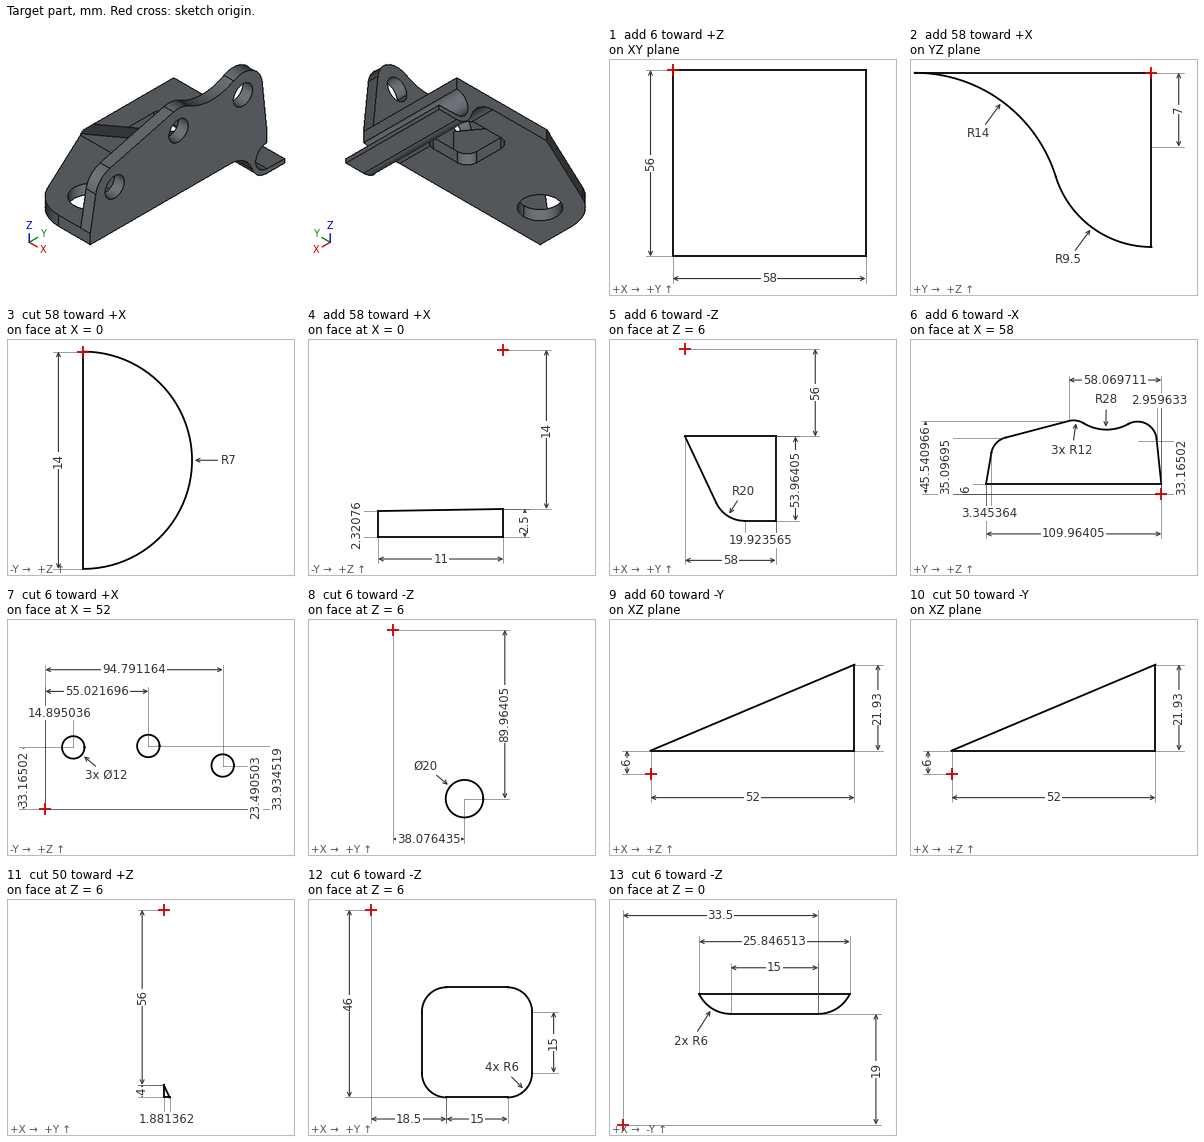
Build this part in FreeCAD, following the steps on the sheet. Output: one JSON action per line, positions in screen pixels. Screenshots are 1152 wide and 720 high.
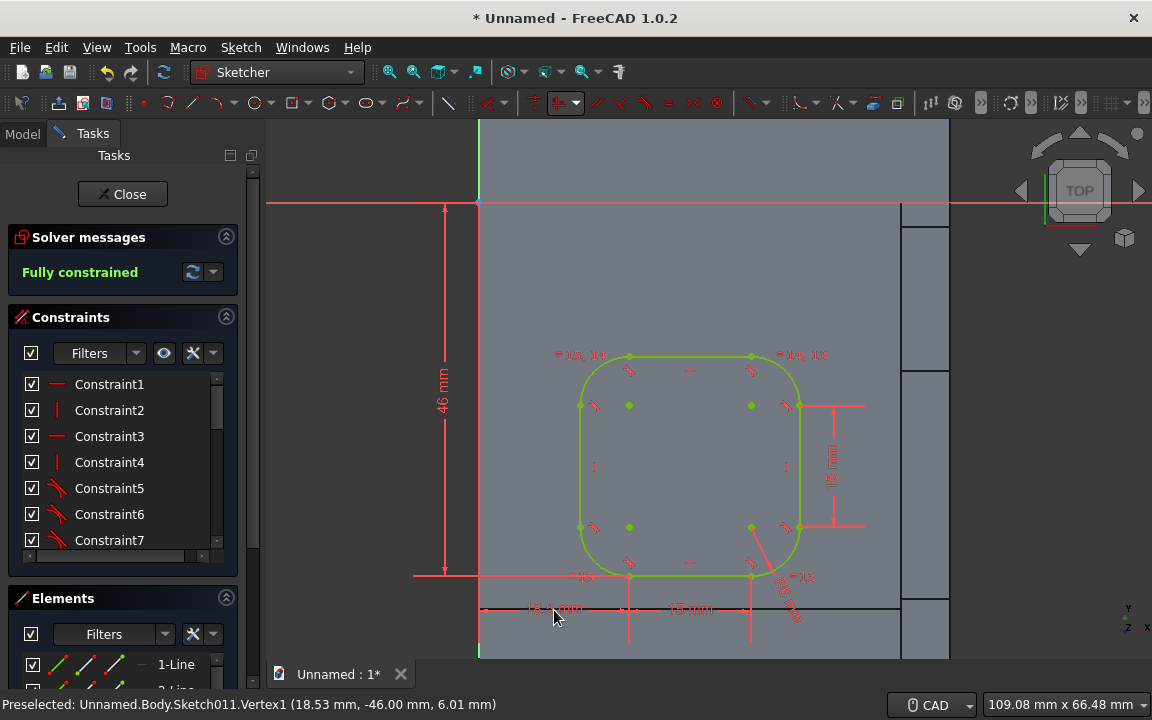
{"action": "left_click", "coordinate": [123, 194]}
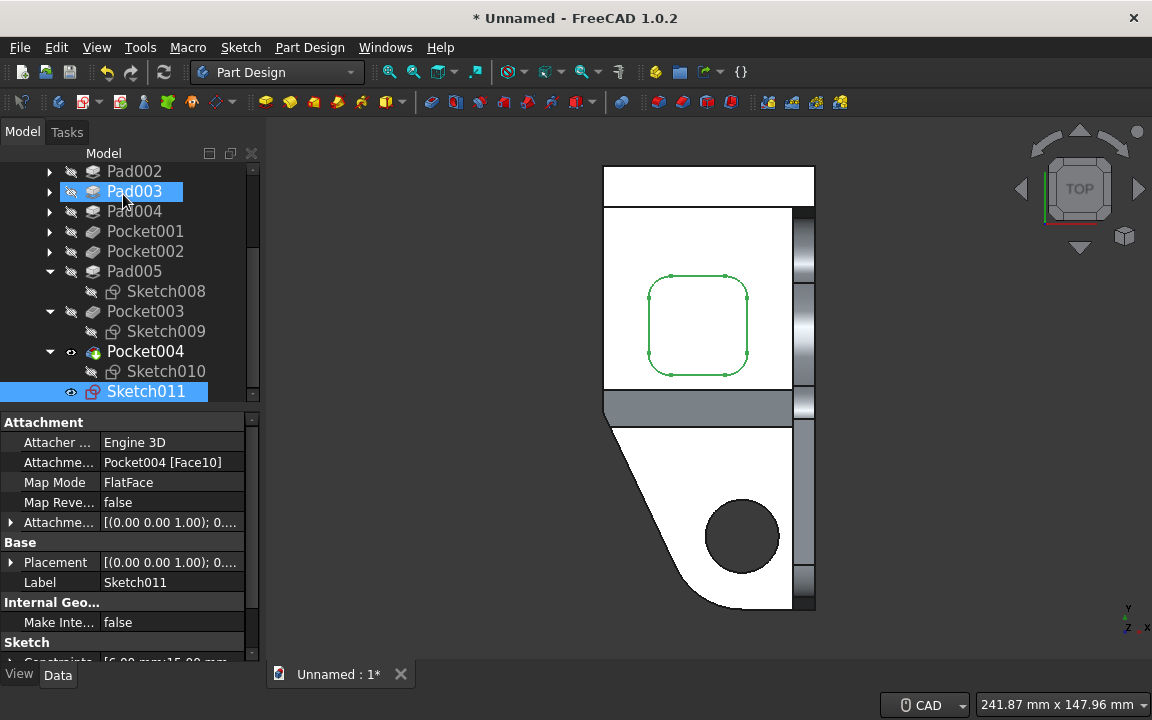
{"action": "left_click", "coordinate": [432, 102]}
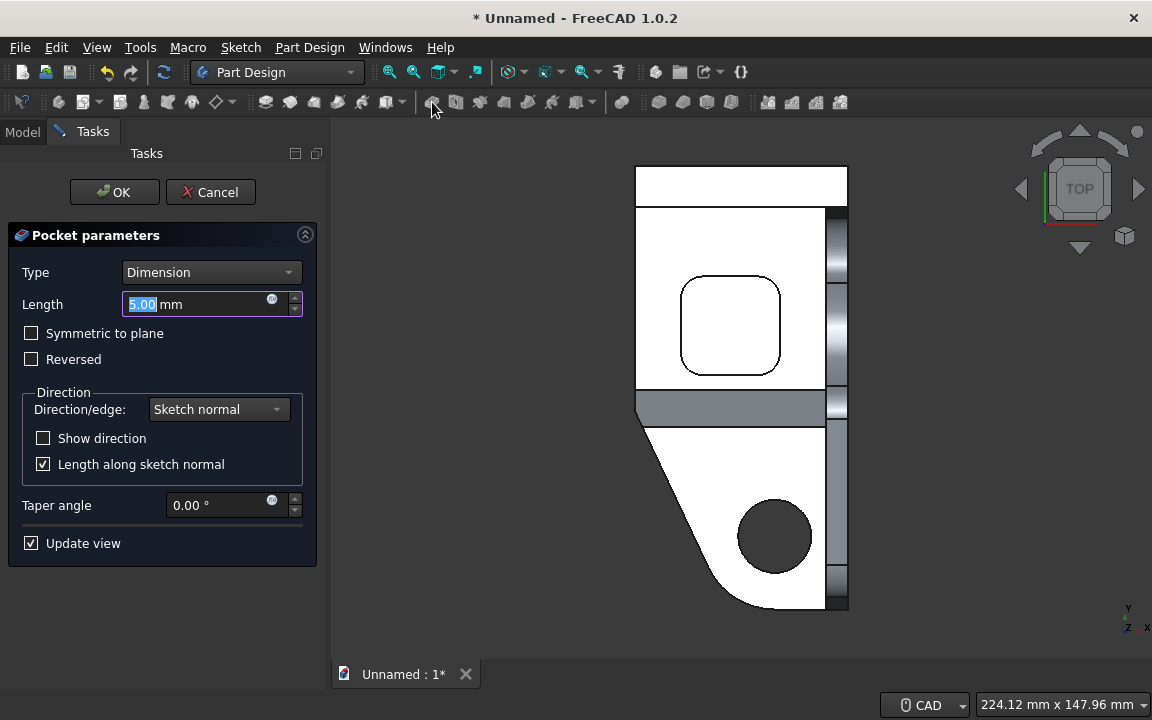
{"action": "type", "text": "6"}
{"action": "key", "text": "Tab"}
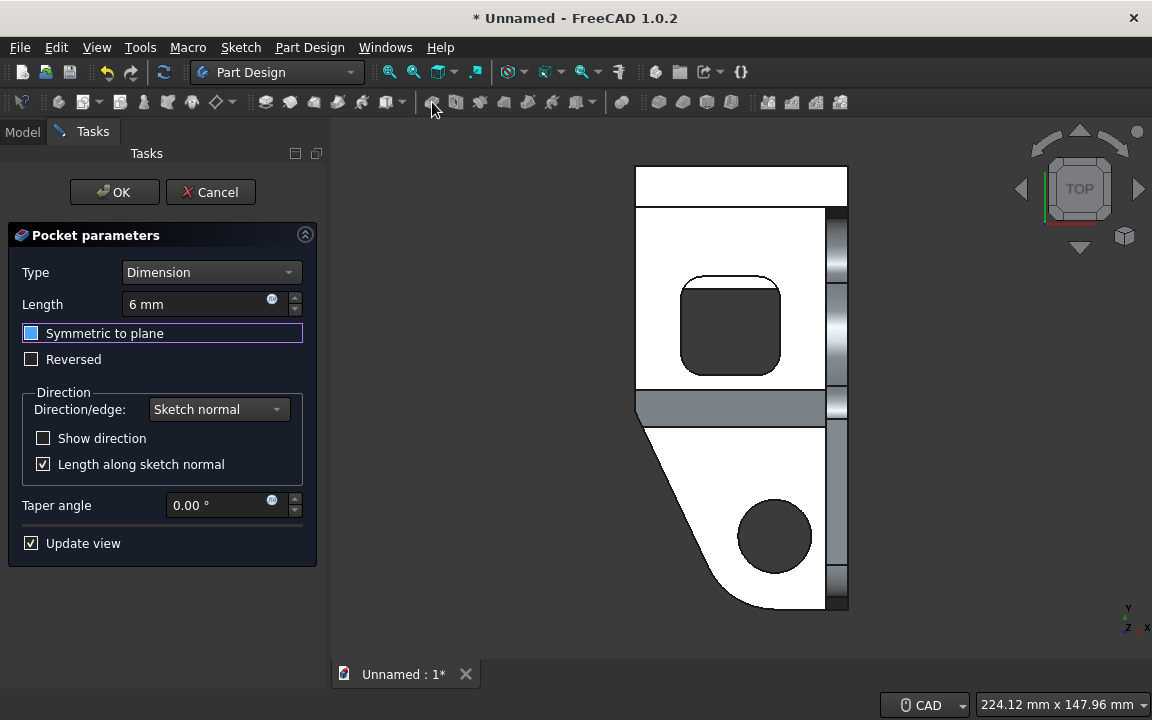
{"action": "left_click", "coordinate": [115, 192]}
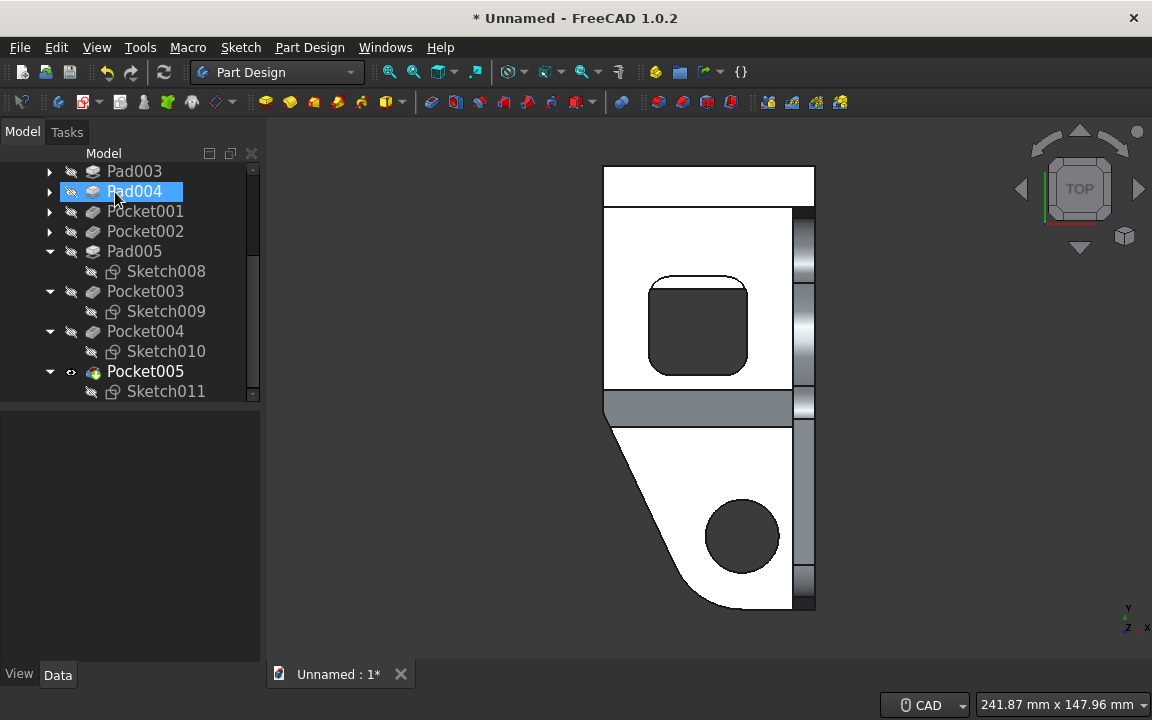
{"action": "key", "text": "5"}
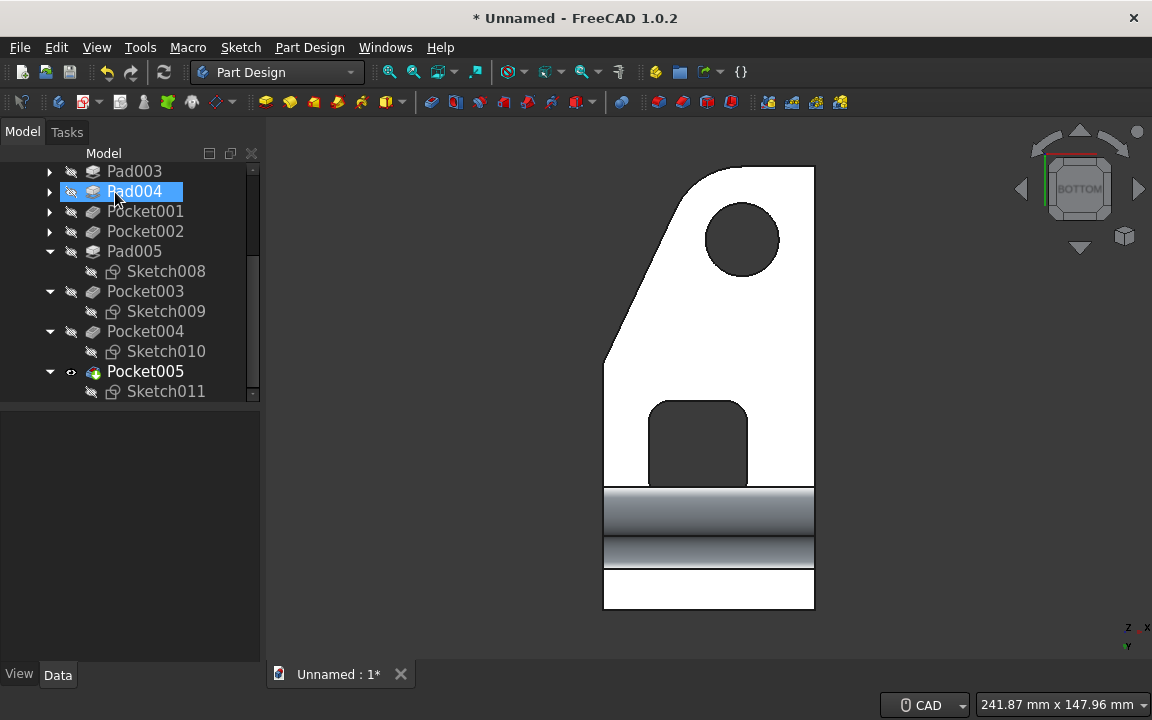
{"action": "left_click", "coordinate": [709, 326]}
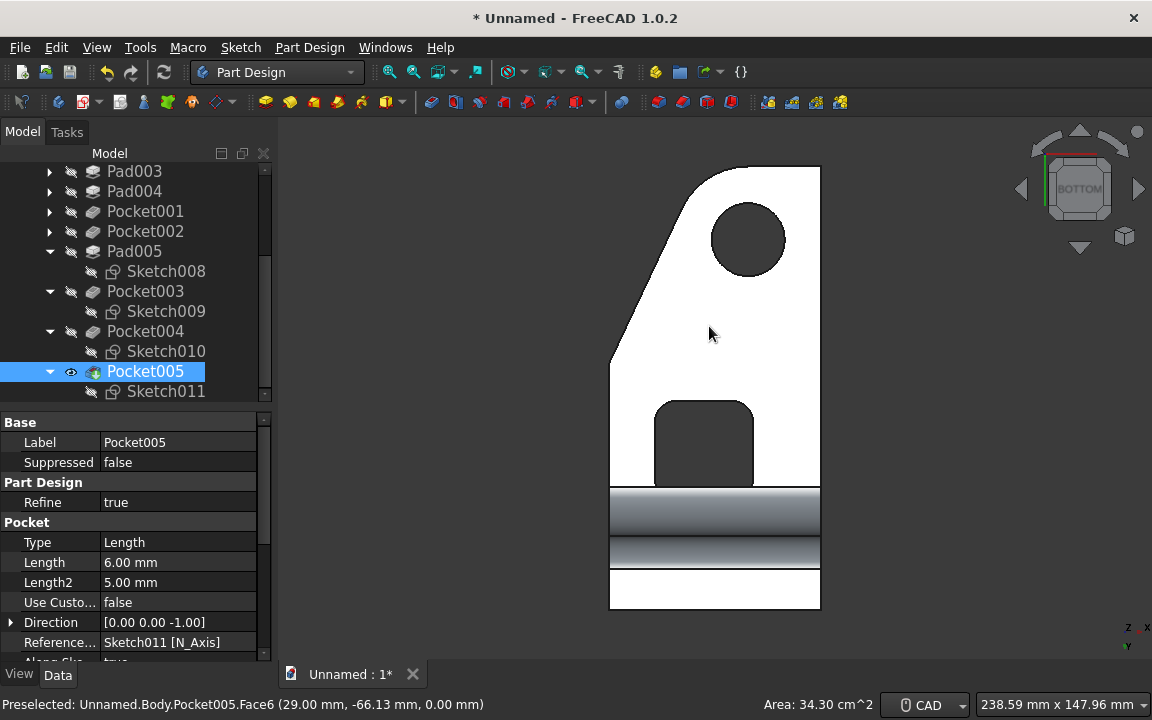
{"action": "left_click", "coordinate": [84, 102]}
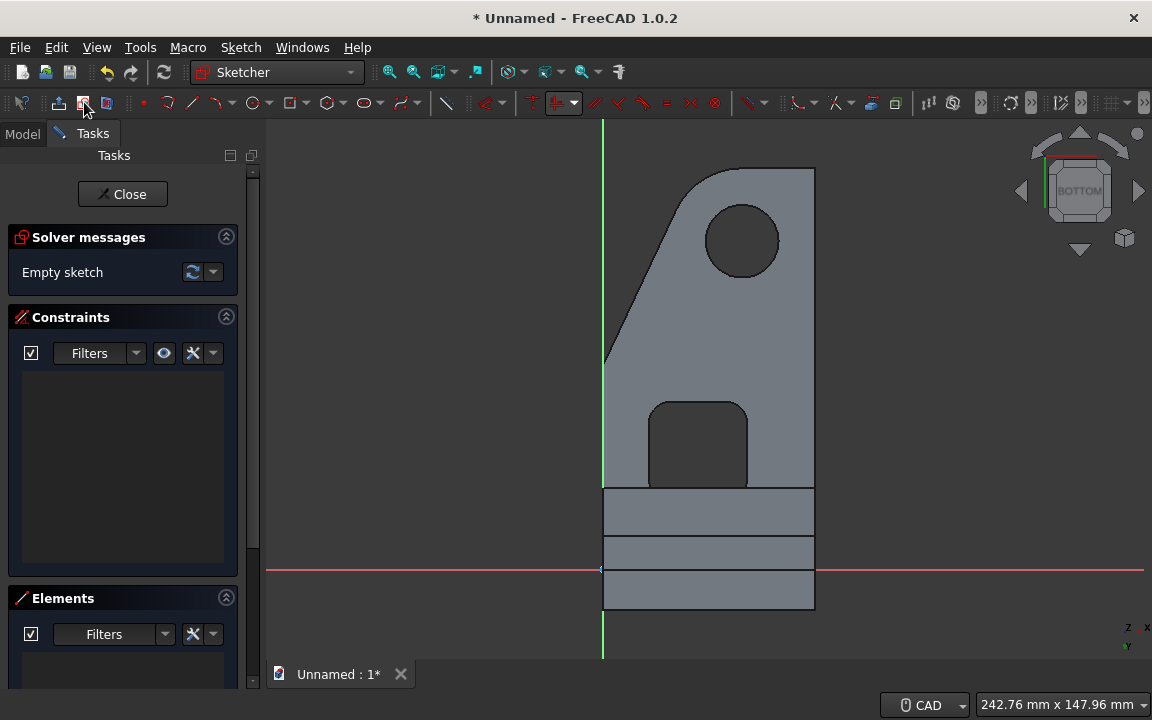
{"action": "left_click", "coordinate": [108, 104]}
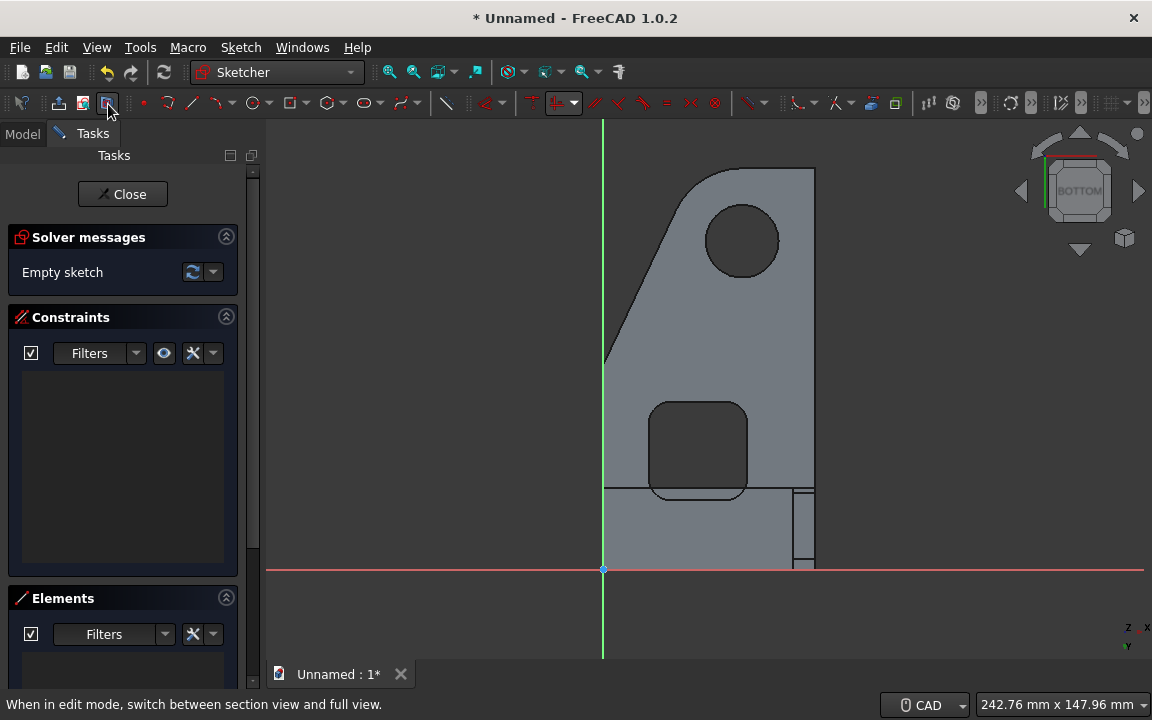
{"action": "scroll", "coordinate": [689, 589], "scroll_direction": "up", "scroll_amount": 6}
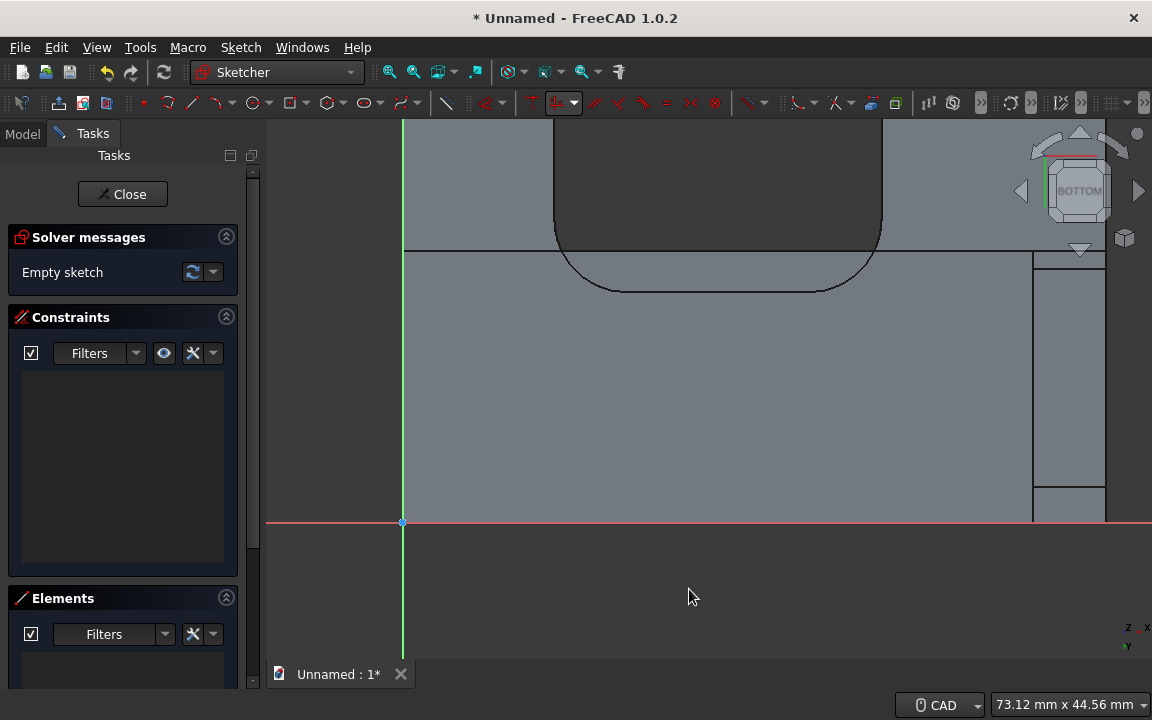
{"action": "key", "text": "g l"}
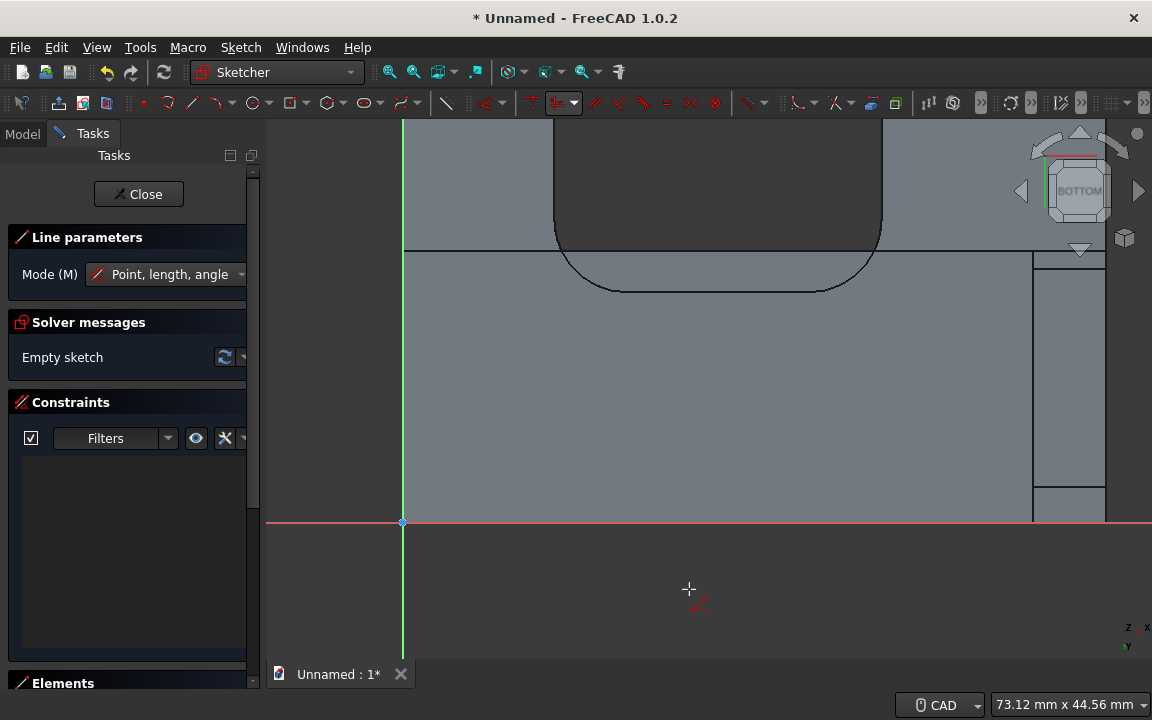
{"action": "left_click", "coordinate": [561, 251]}
{"action": "left_click", "coordinate": [875, 251]}